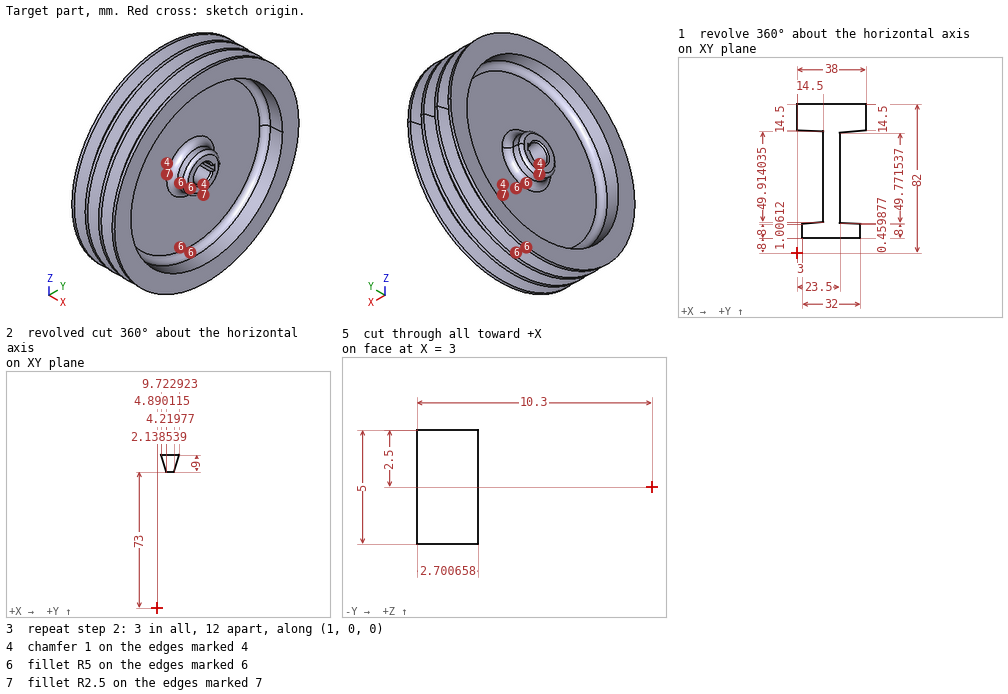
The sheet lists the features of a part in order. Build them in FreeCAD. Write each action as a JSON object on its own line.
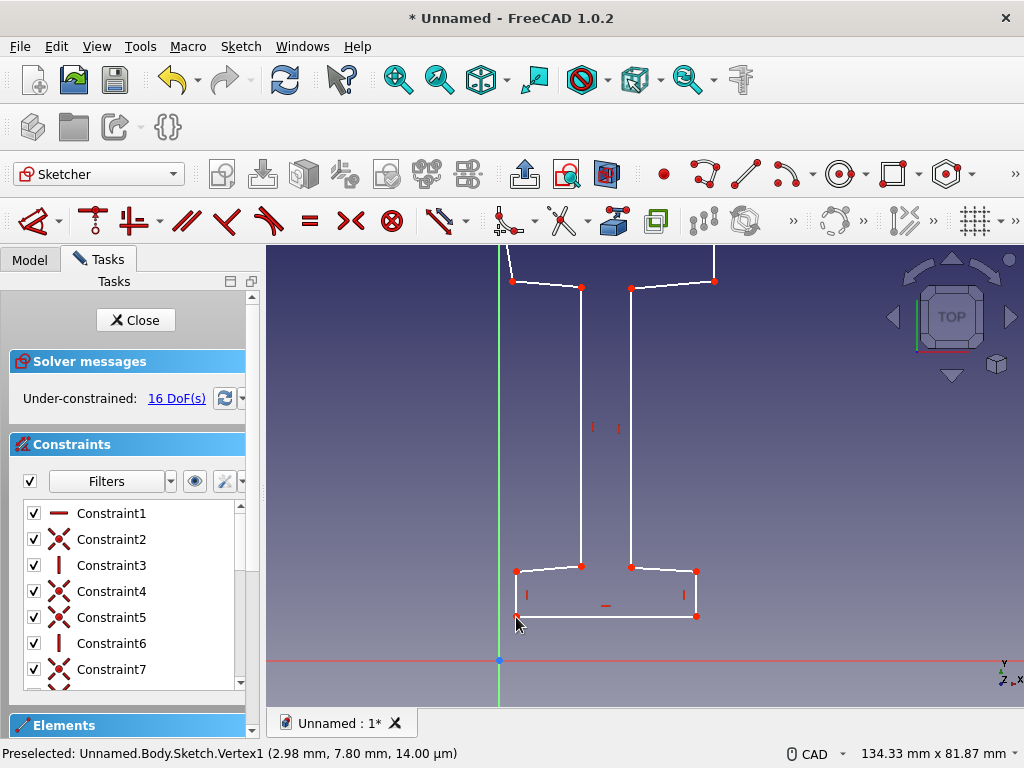
{"action": "scroll", "coordinate": [516, 571], "scroll_direction": "down", "scroll_amount": 2}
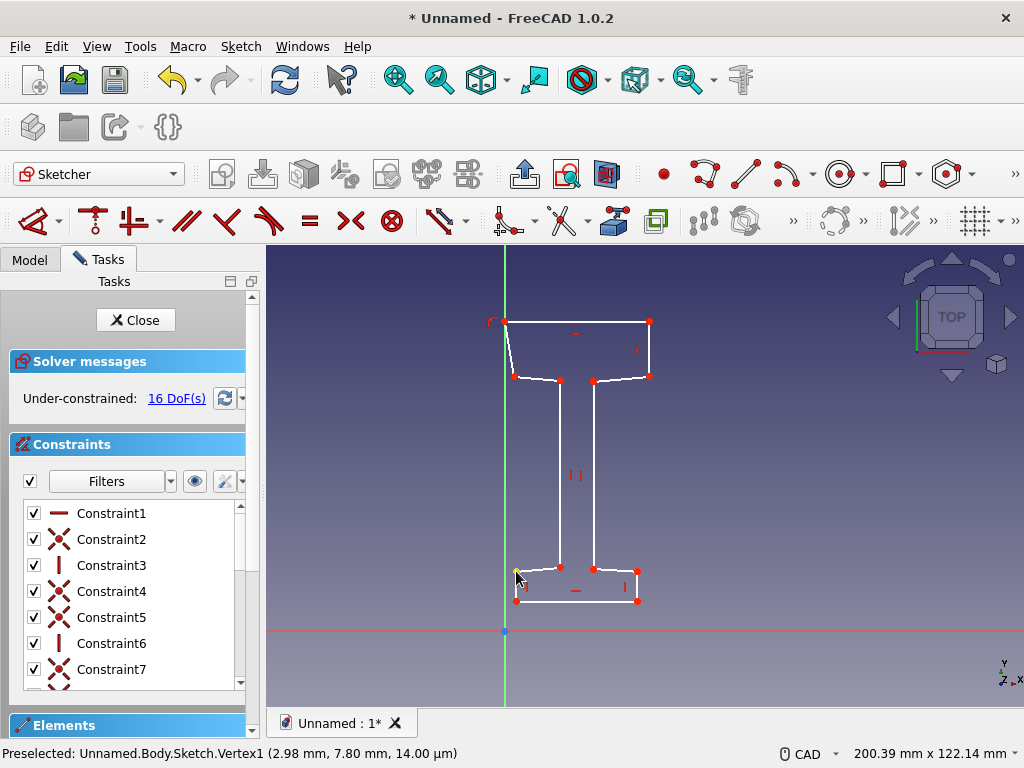
{"action": "scroll", "coordinate": [511, 361], "scroll_direction": "up", "scroll_amount": 4}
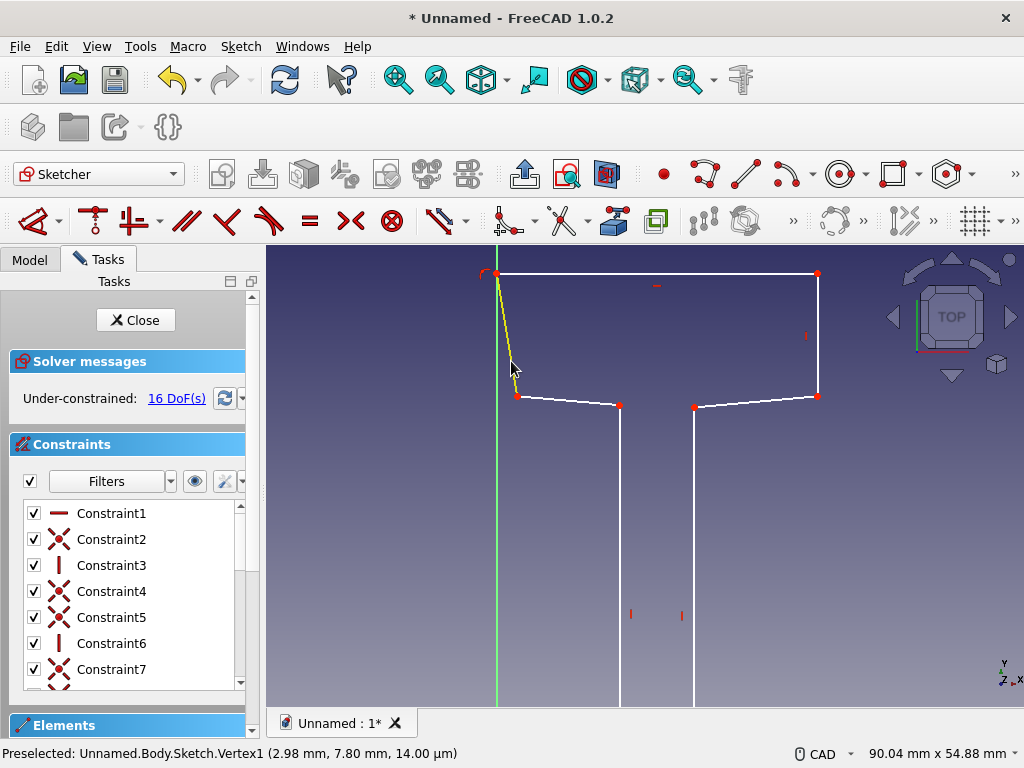
{"action": "left_click", "coordinate": [511, 360]}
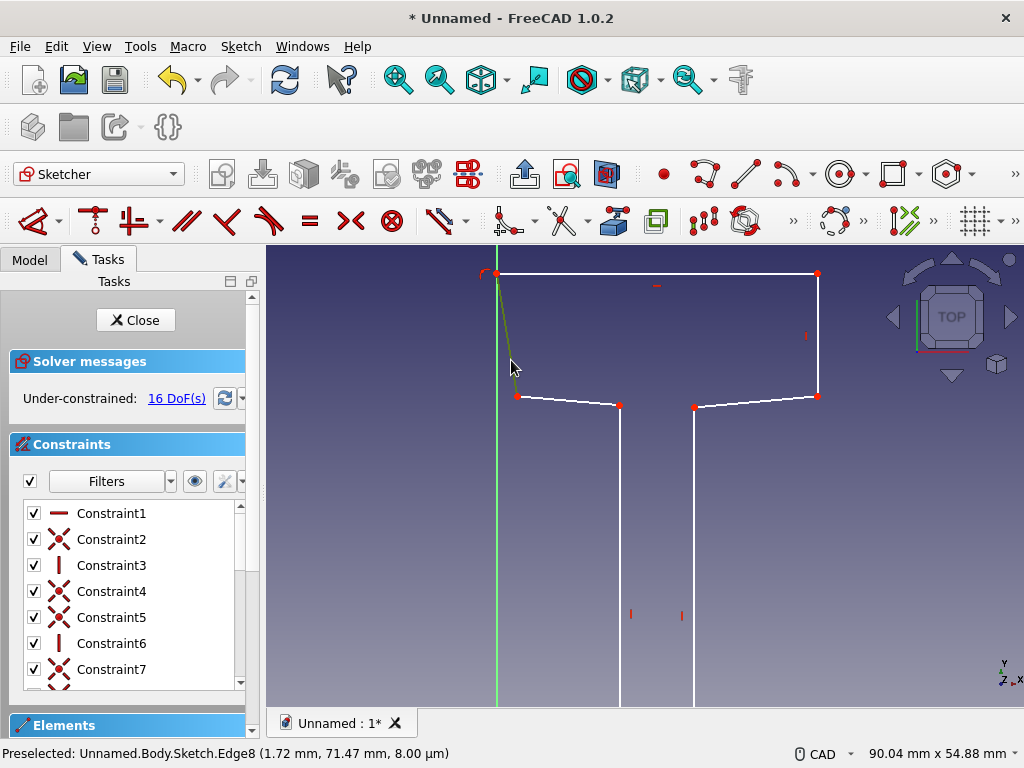
{"action": "key", "text": "v"}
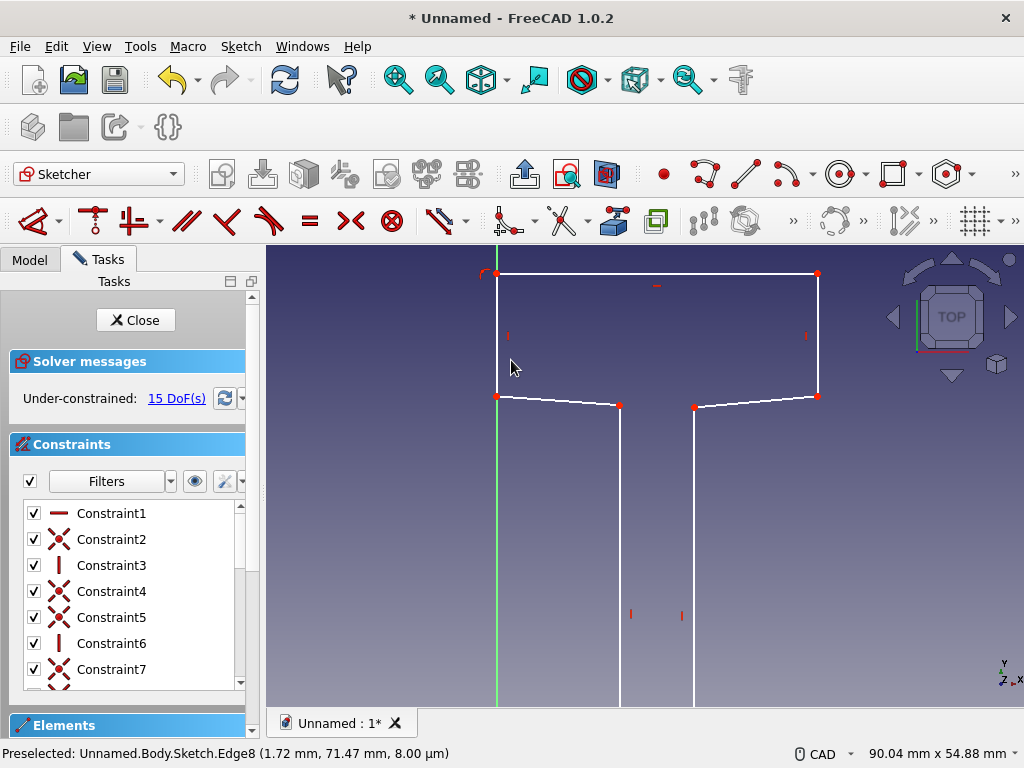
{"action": "scroll", "coordinate": [511, 361], "scroll_direction": "down", "scroll_amount": 4}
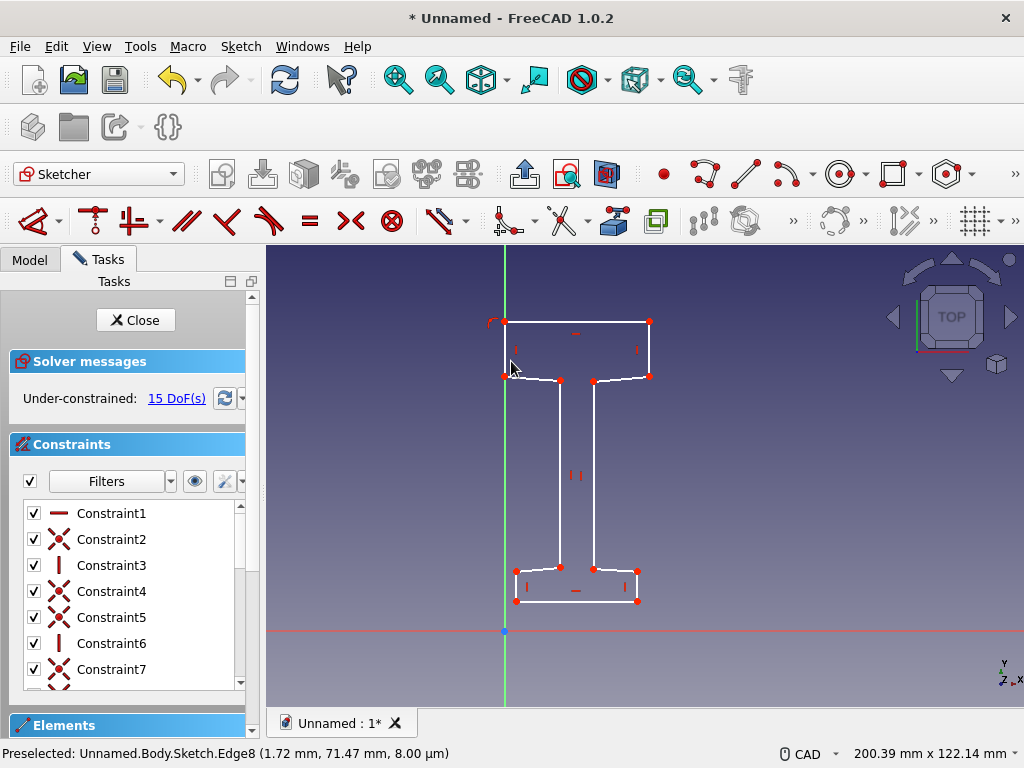
{"action": "scroll", "coordinate": [637, 593], "scroll_direction": "up", "scroll_amount": 3}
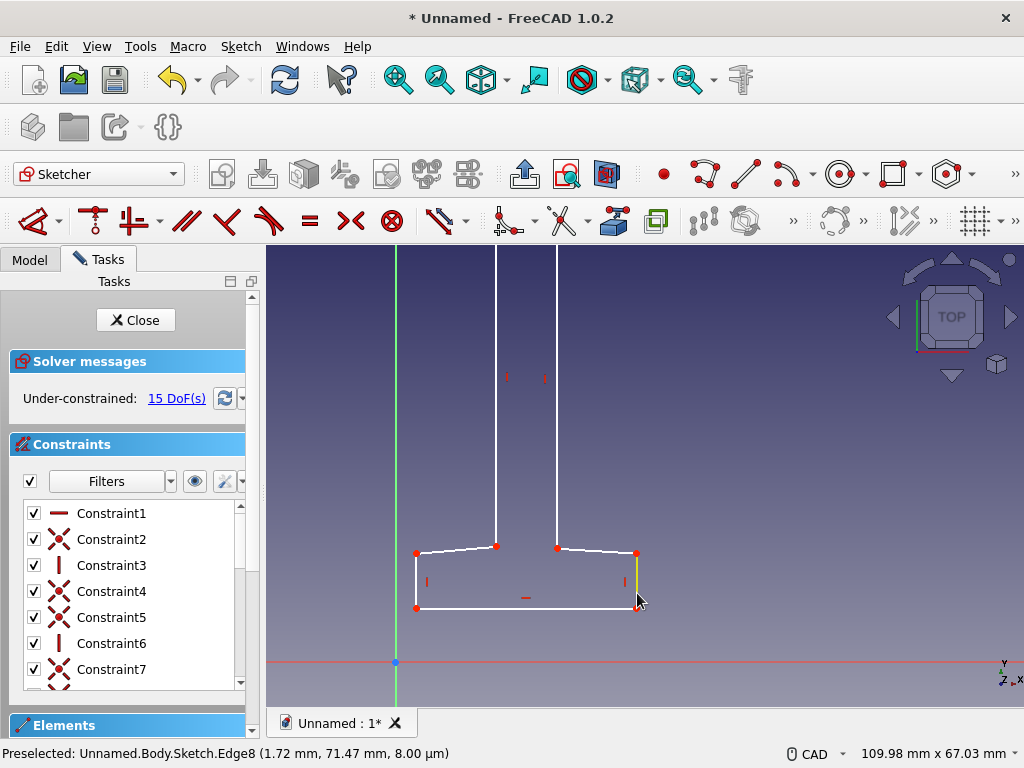
{"action": "left_click", "coordinate": [637, 592]}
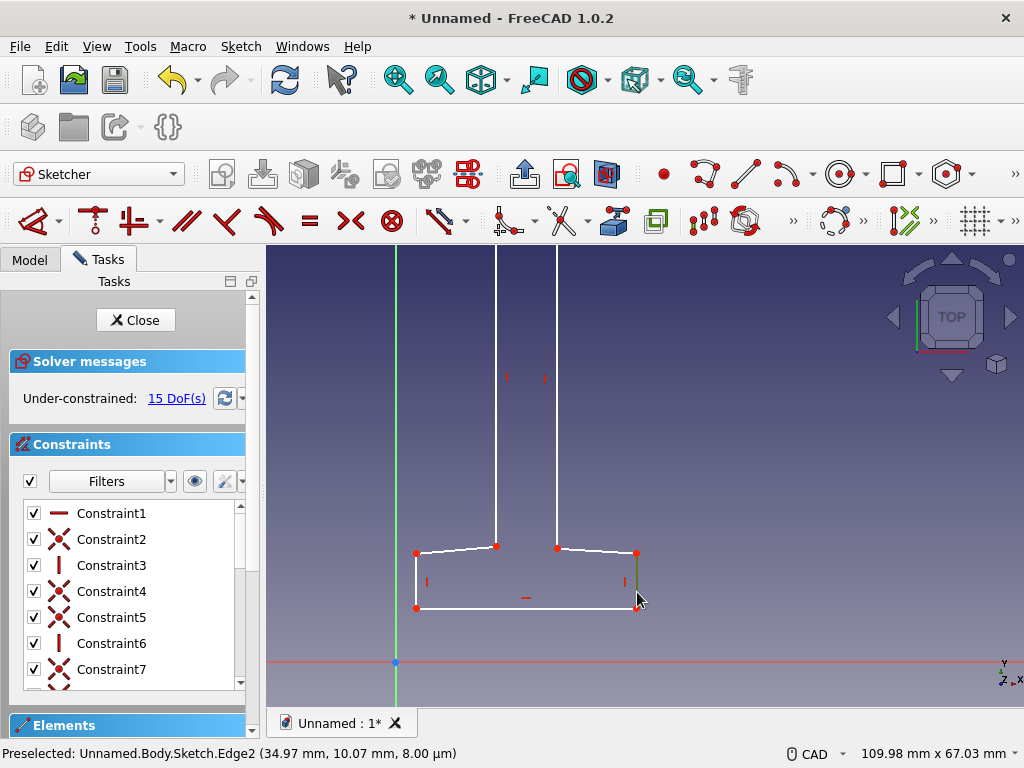
{"action": "left_click", "coordinate": [58, 222]}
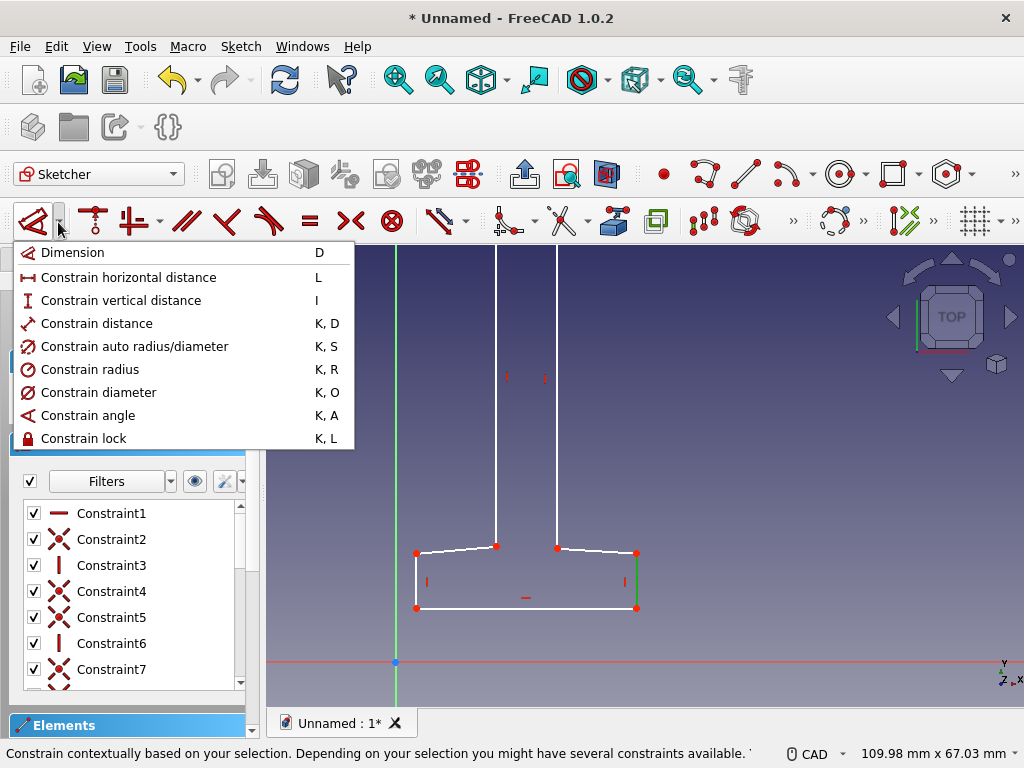
{"action": "left_click", "coordinate": [184, 300]}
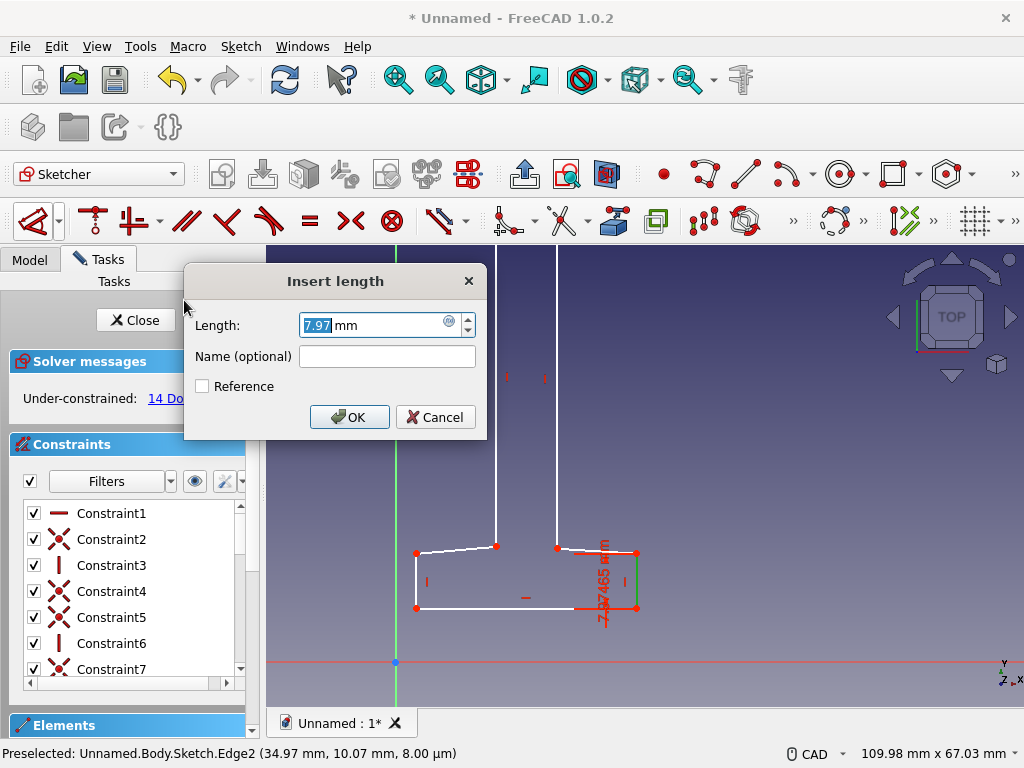
{"action": "type", "text": "8"}
{"action": "key", "text": "Return"}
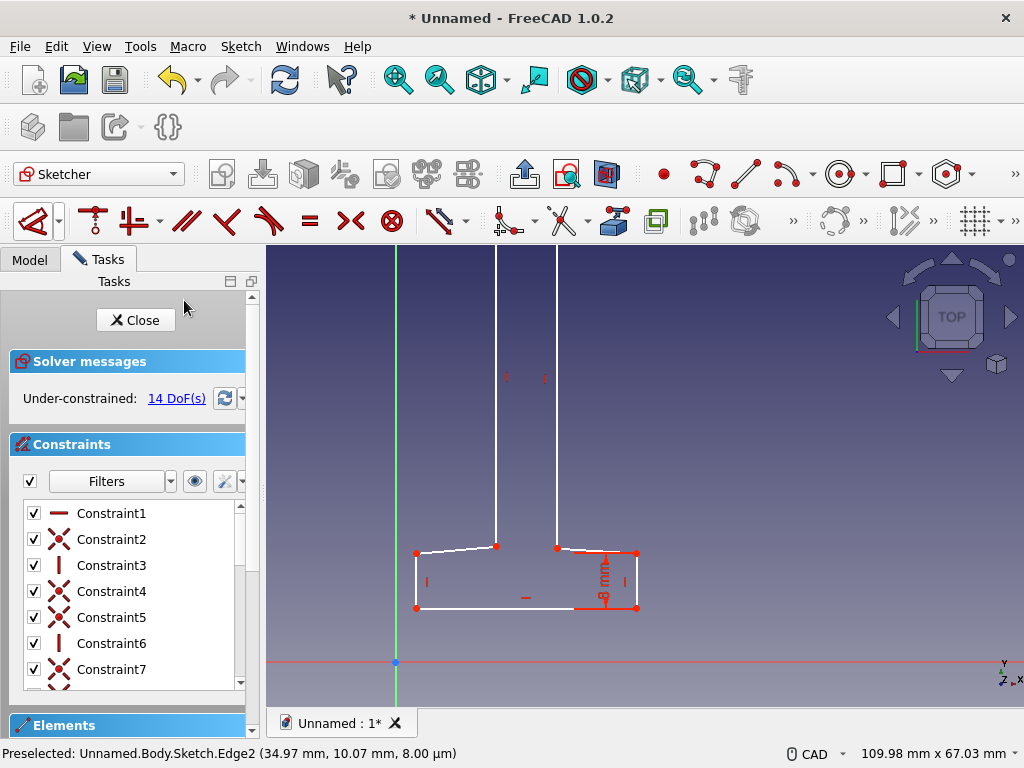
{"action": "left_click", "coordinate": [416, 570]}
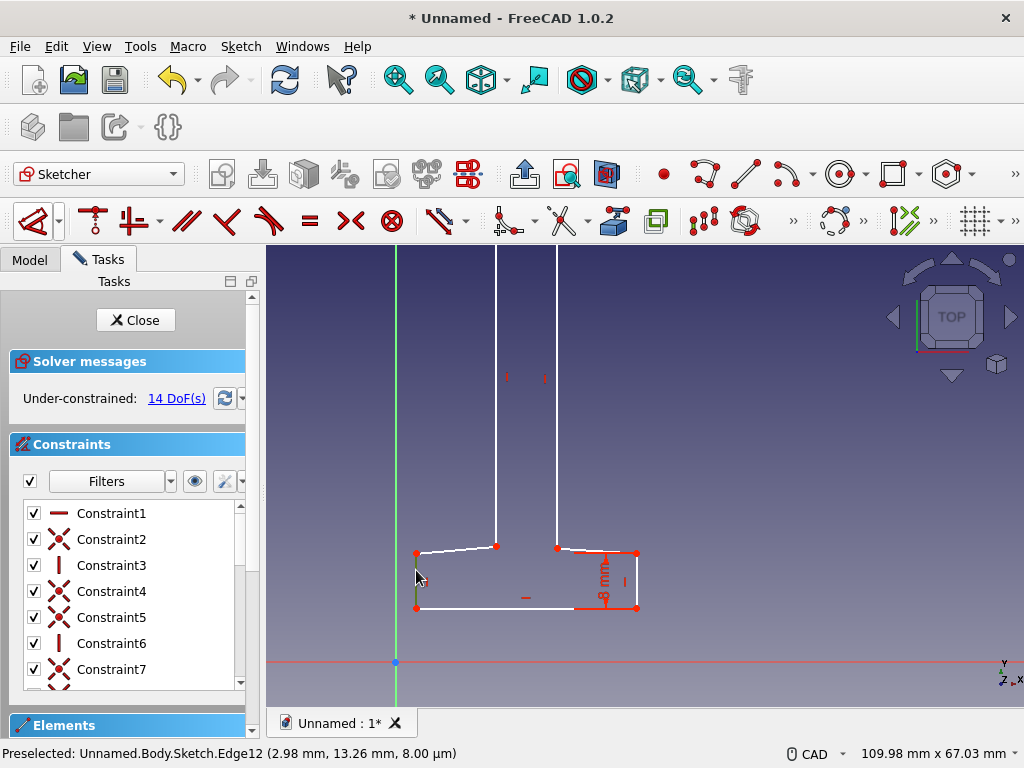
{"action": "left_click", "coordinate": [58, 222]}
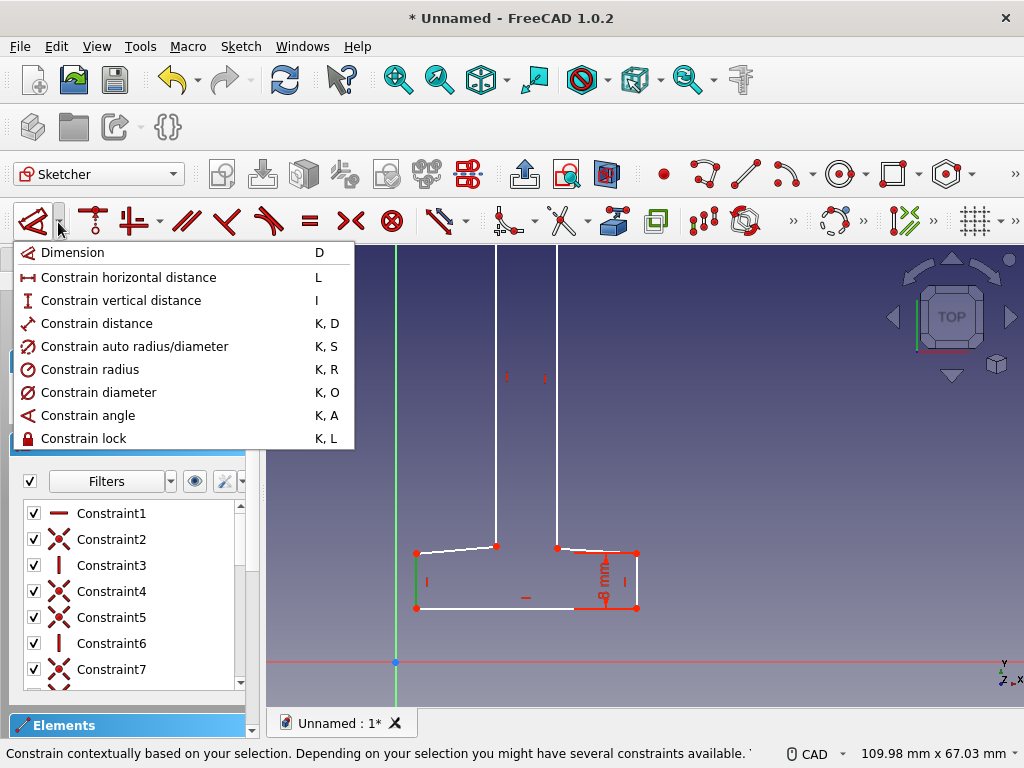
{"action": "left_click", "coordinate": [184, 300]}